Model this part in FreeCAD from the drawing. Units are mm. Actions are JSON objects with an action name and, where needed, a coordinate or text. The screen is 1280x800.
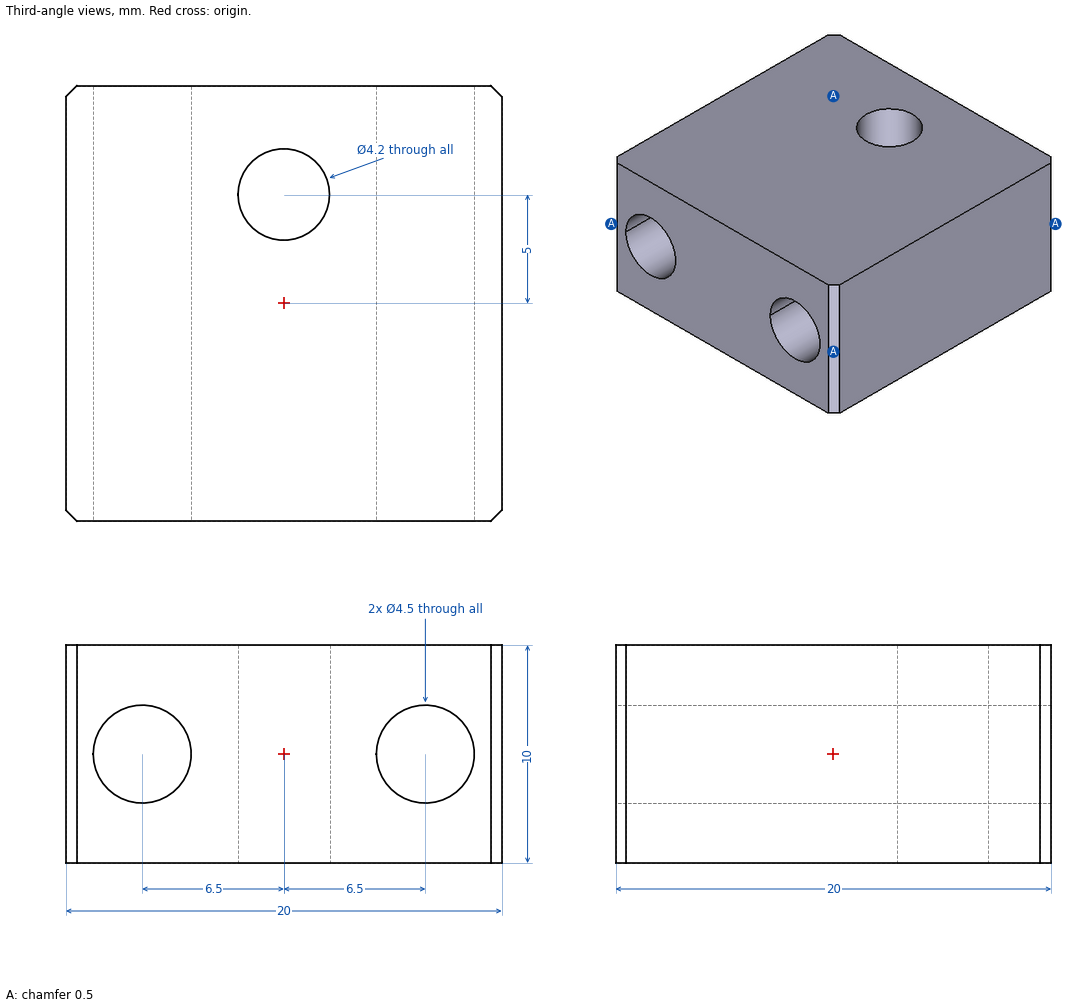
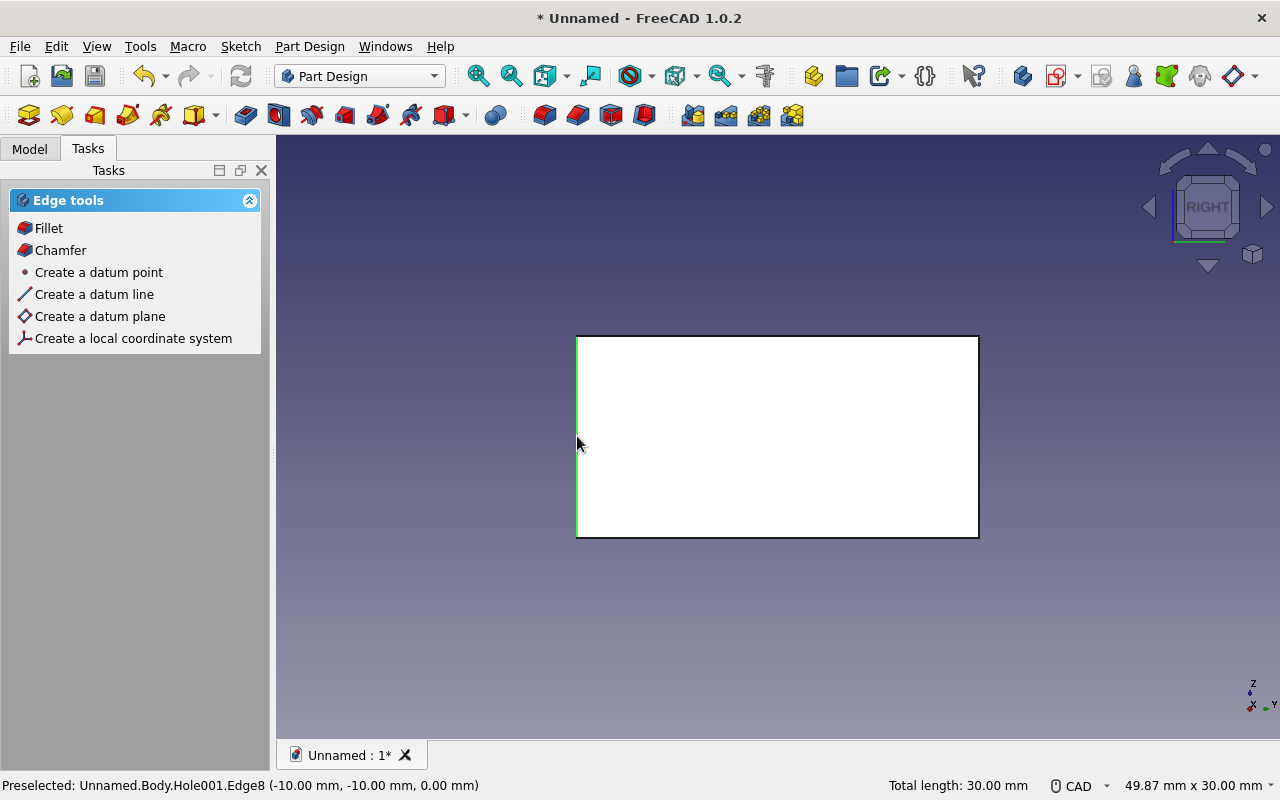
{"action": "left_click", "coordinate": [979, 436], "text": "ctrl"}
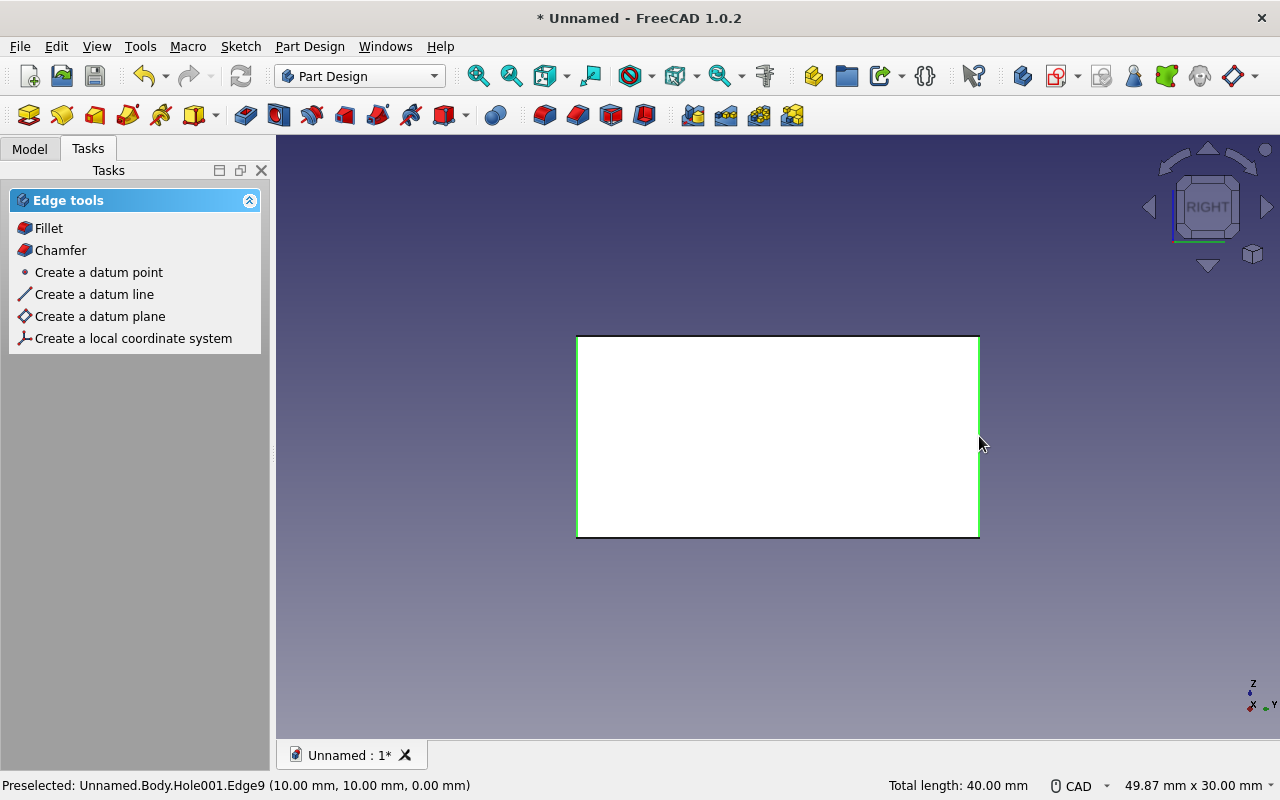
{"action": "left_click", "coordinate": [578, 116]}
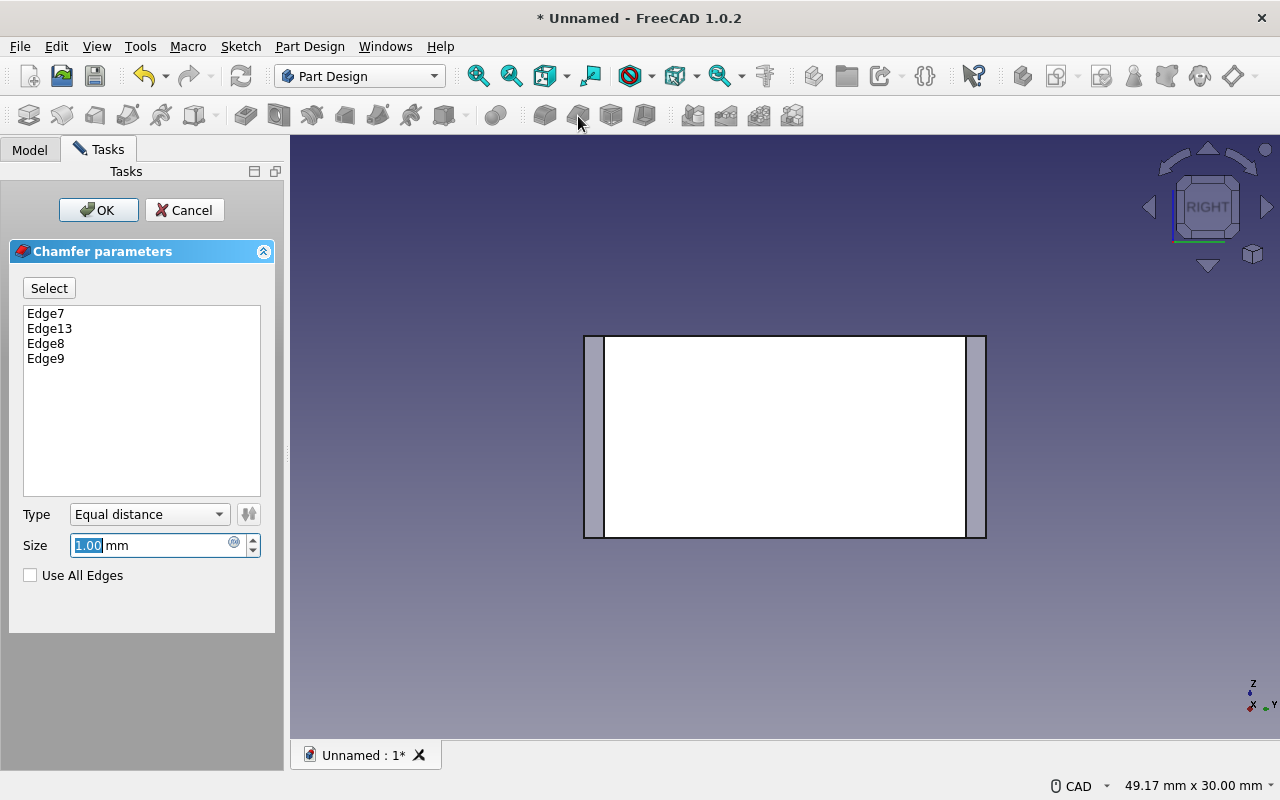
{"action": "type", "text": "0.5"}
{"action": "key", "text": "Tab"}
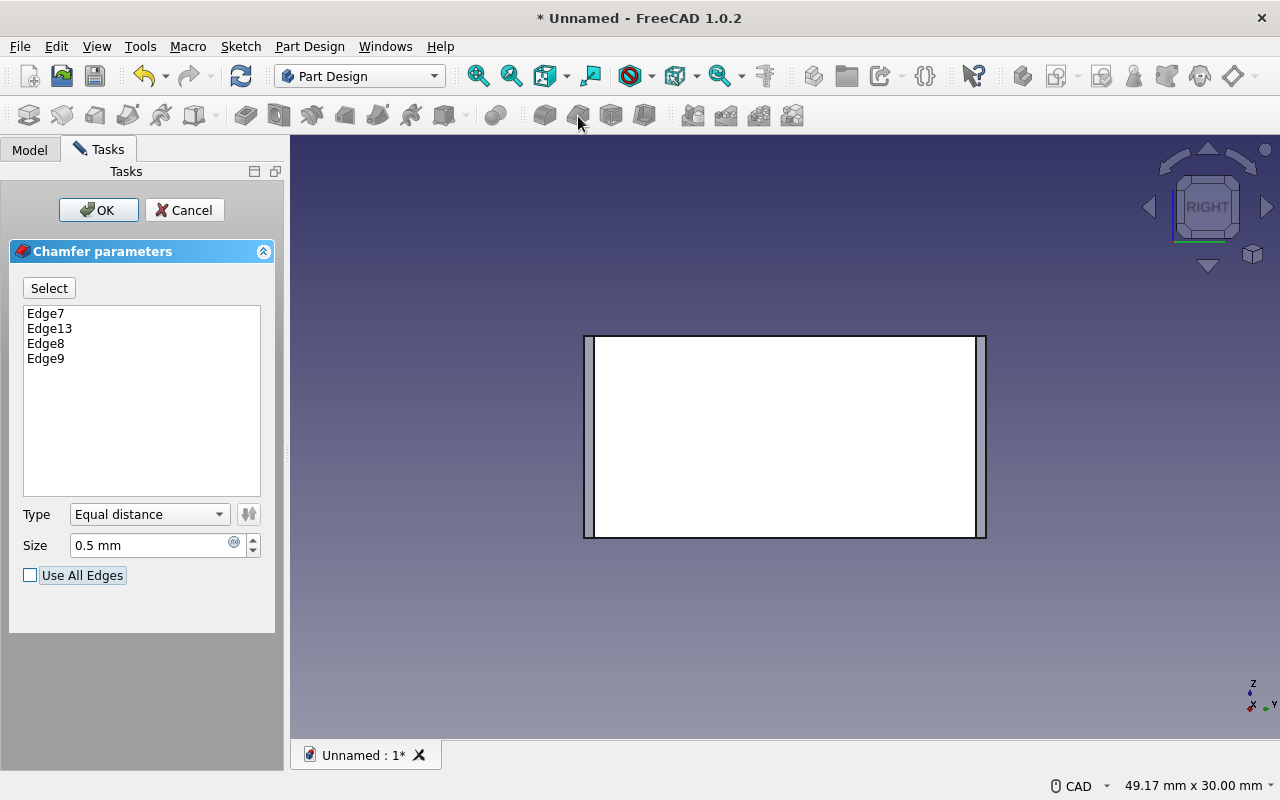
{"action": "left_click", "coordinate": [99, 210]}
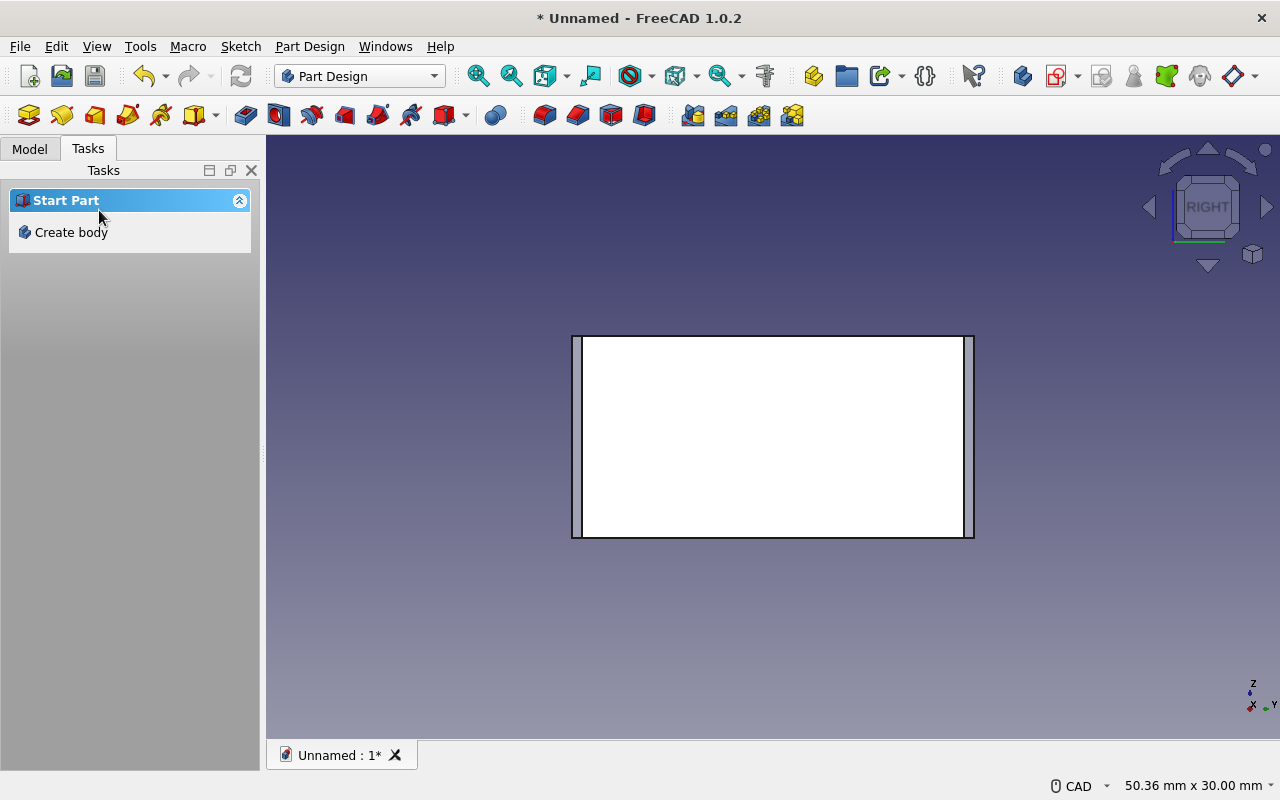
{"action": "key", "text": "0"}